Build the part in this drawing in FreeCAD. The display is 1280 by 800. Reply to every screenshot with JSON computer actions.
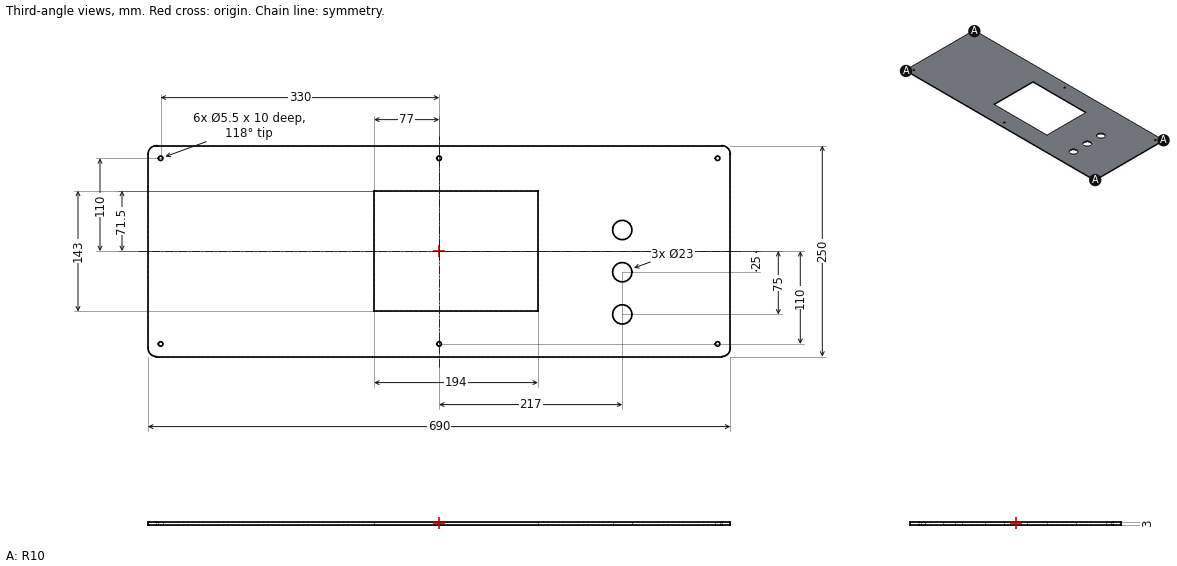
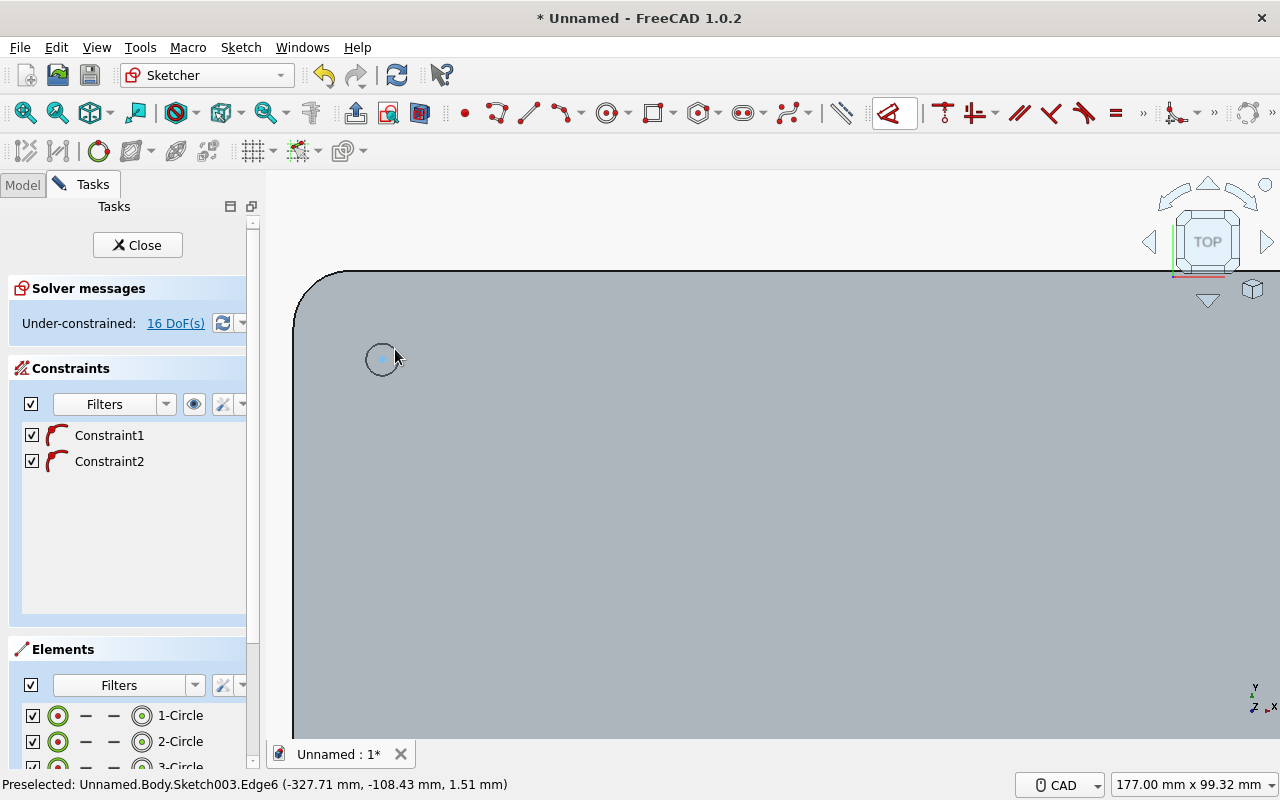
{"action": "left_click", "coordinate": [394, 348]}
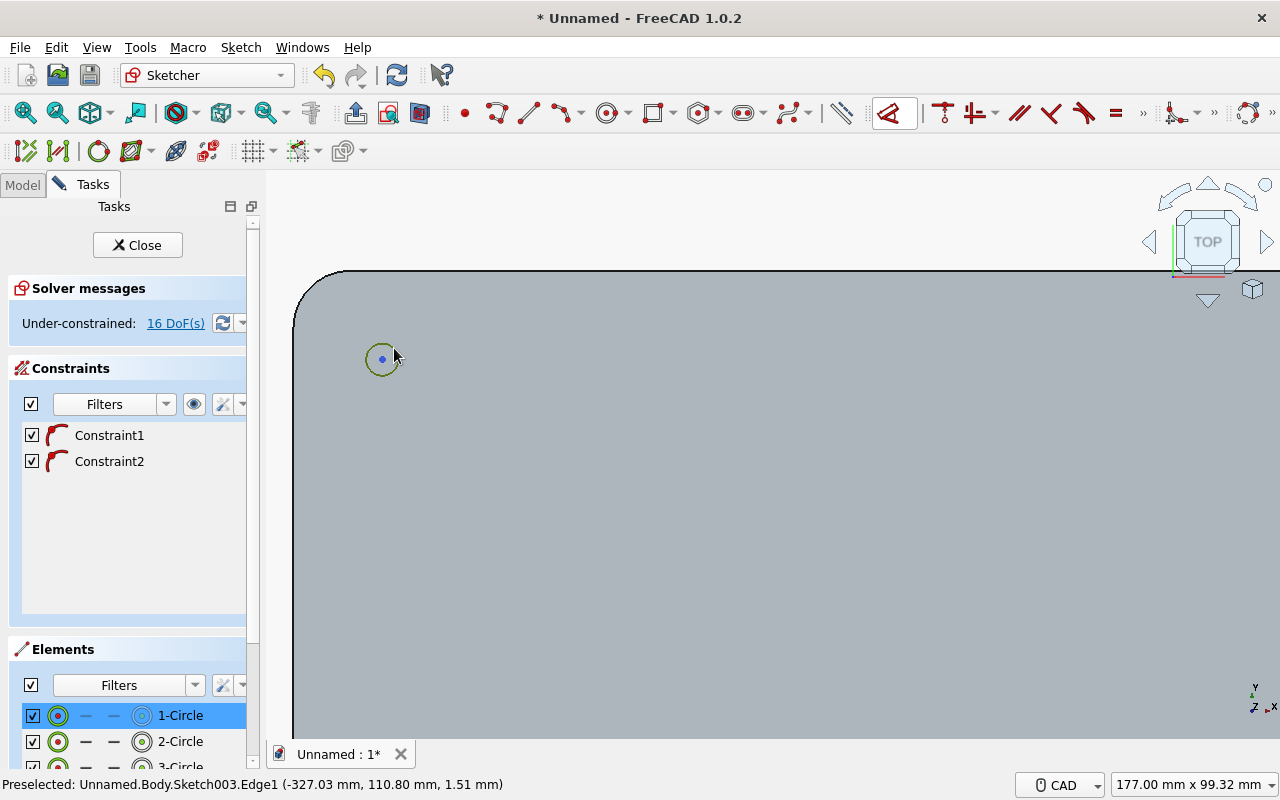
{"action": "scroll", "coordinate": [395, 349], "scroll_direction": "down", "scroll_amount": 9}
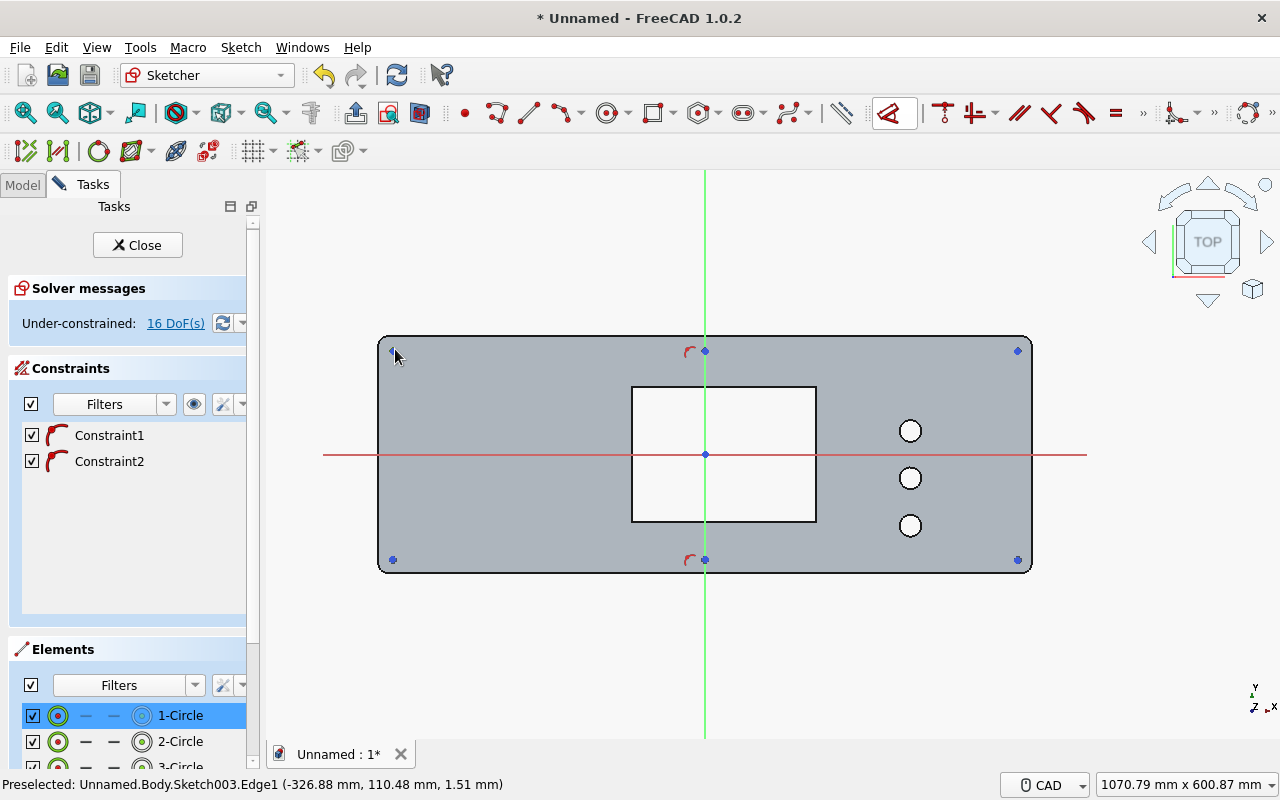
{"action": "scroll", "coordinate": [707, 349], "scroll_direction": "up", "scroll_amount": 10}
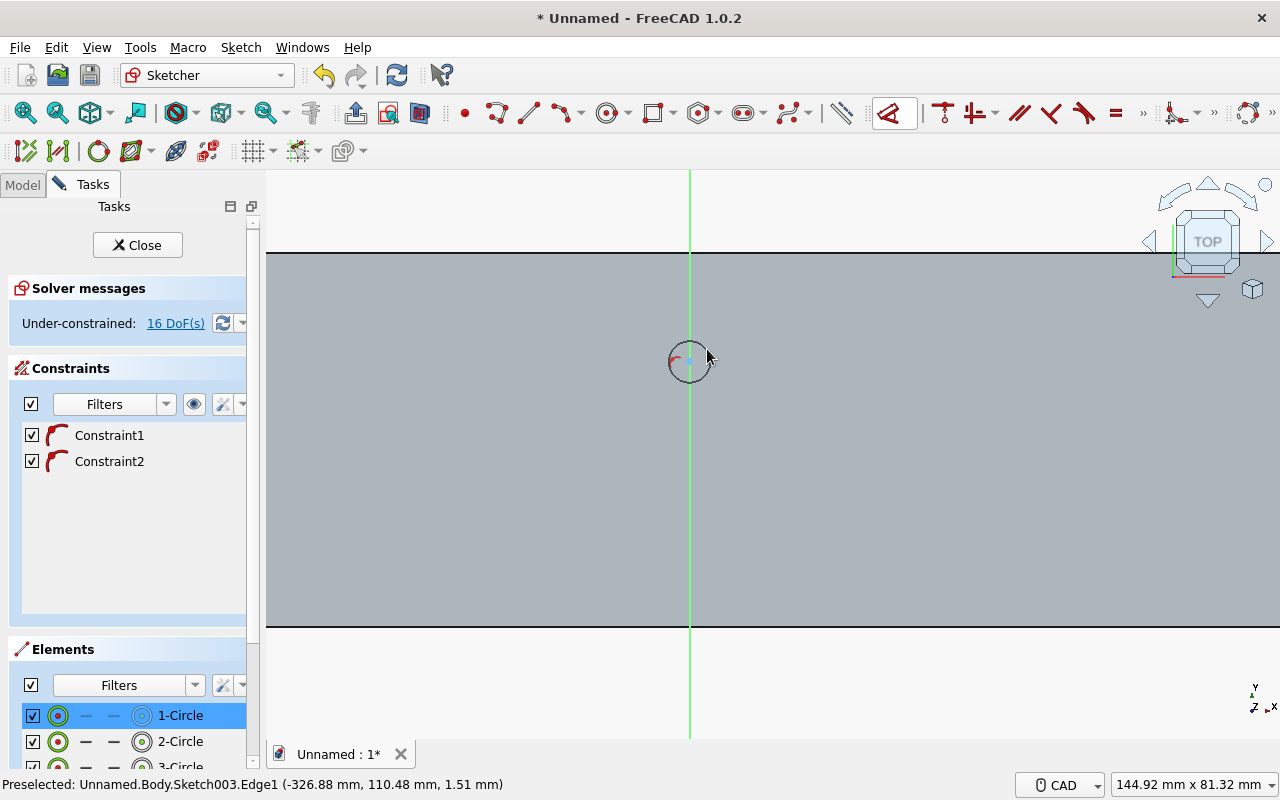
{"action": "left_click", "coordinate": [704, 347]}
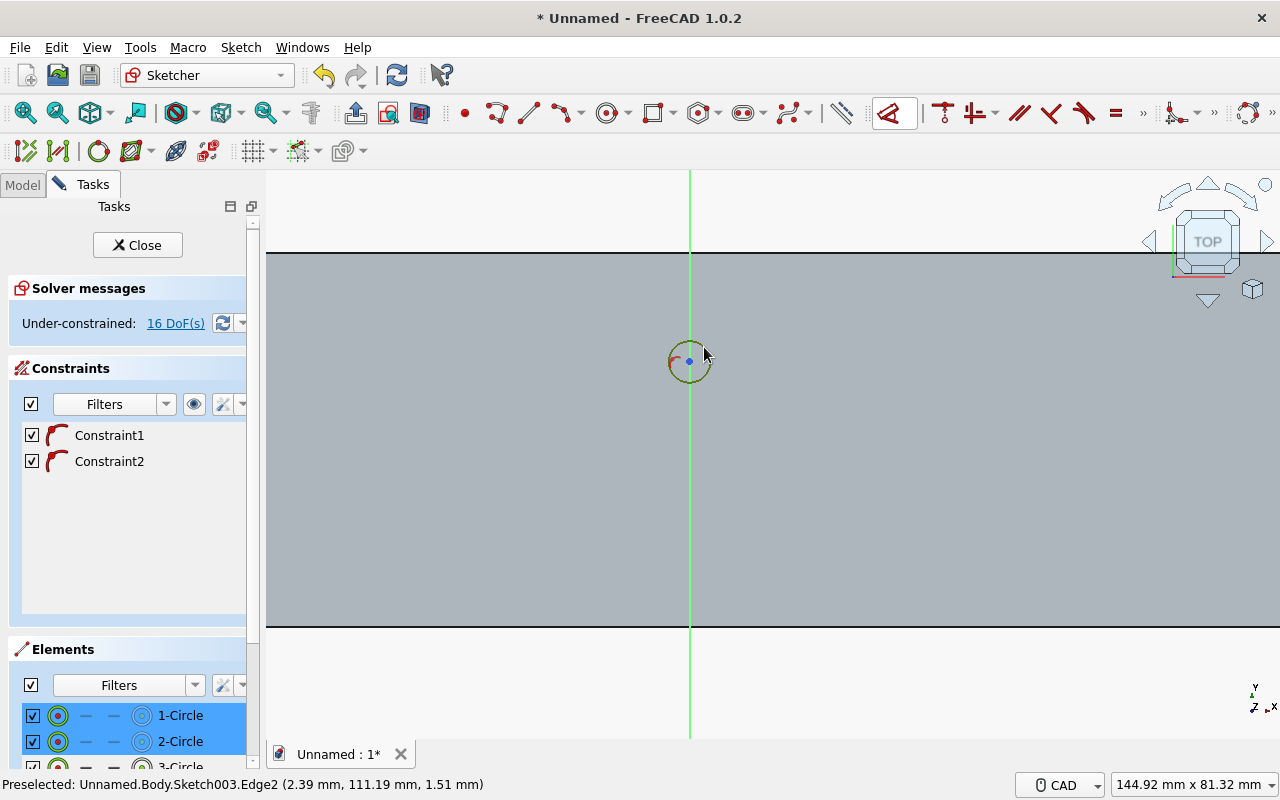
{"action": "scroll", "coordinate": [707, 349], "scroll_direction": "down", "scroll_amount": 10}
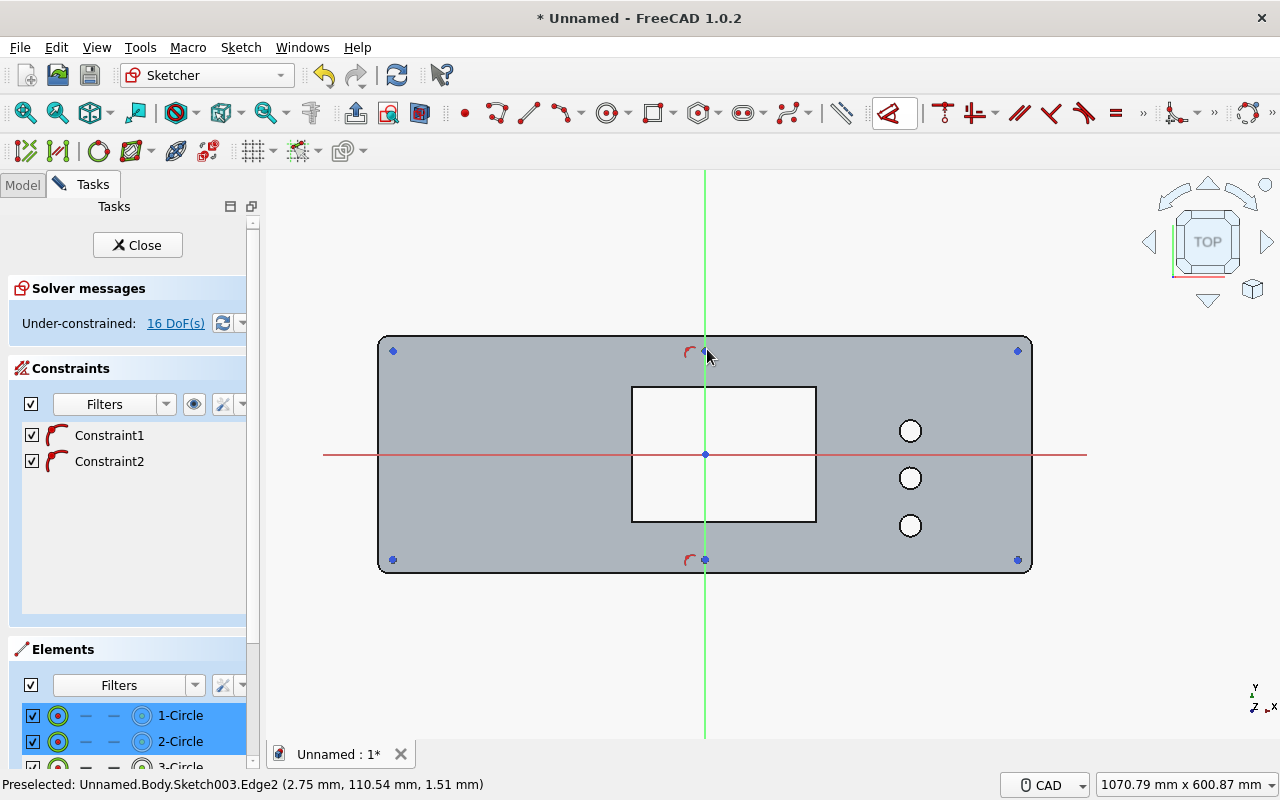
{"action": "scroll", "coordinate": [1020, 349], "scroll_direction": "up", "scroll_amount": 9}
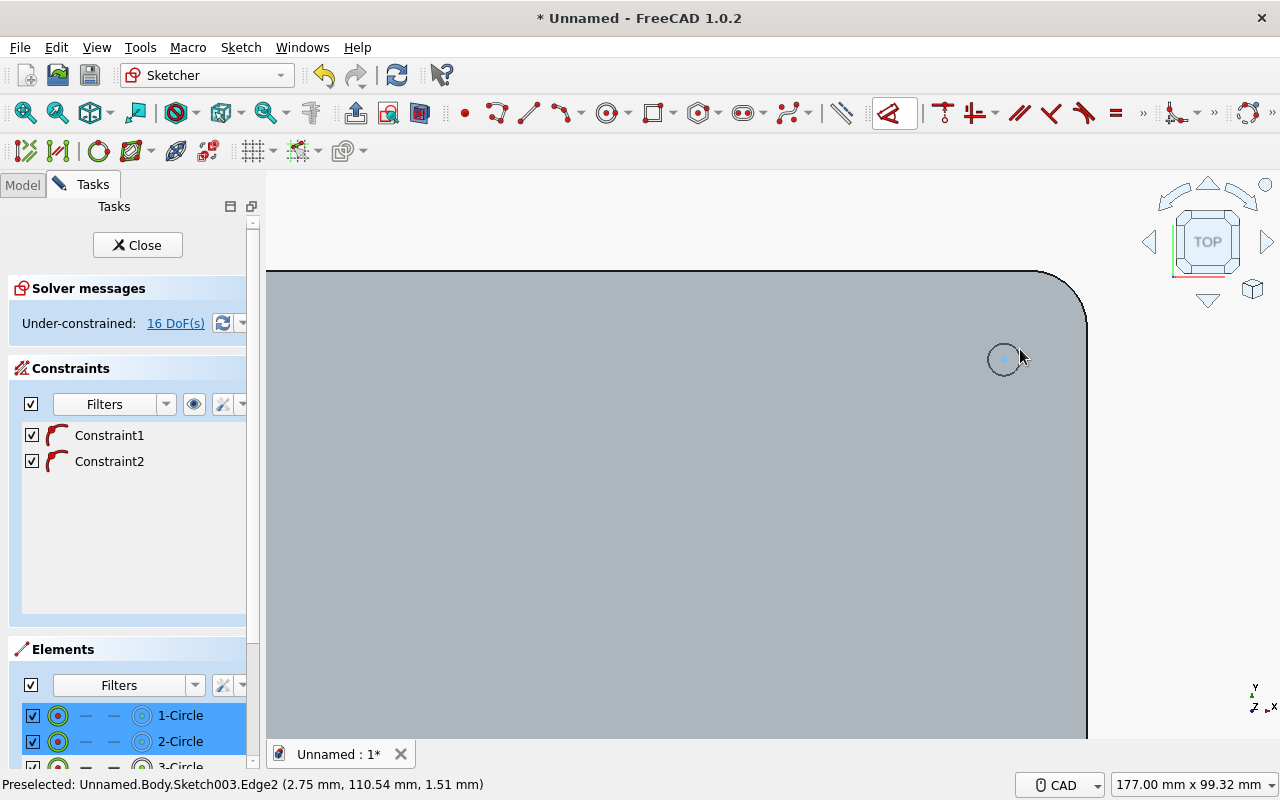
{"action": "left_click", "coordinate": [1015, 348]}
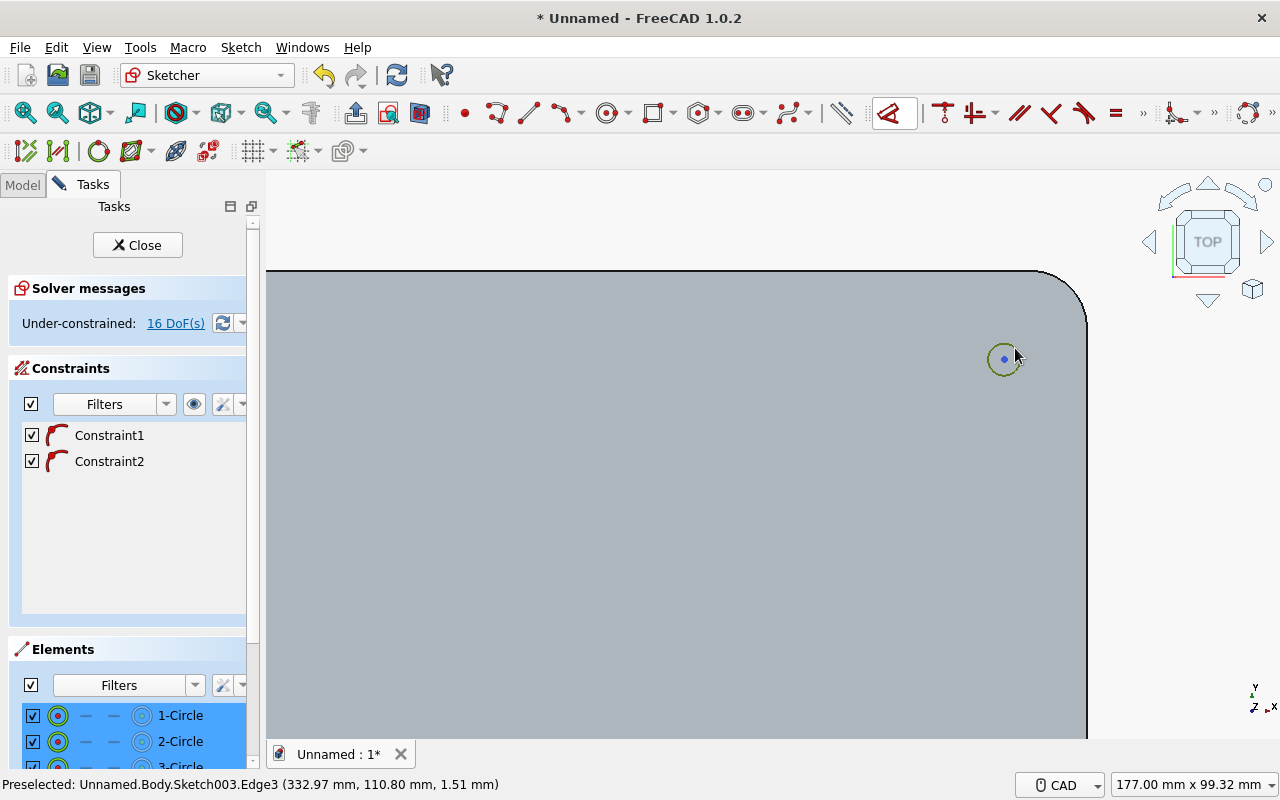
{"action": "scroll", "coordinate": [1020, 349], "scroll_direction": "down", "scroll_amount": 9}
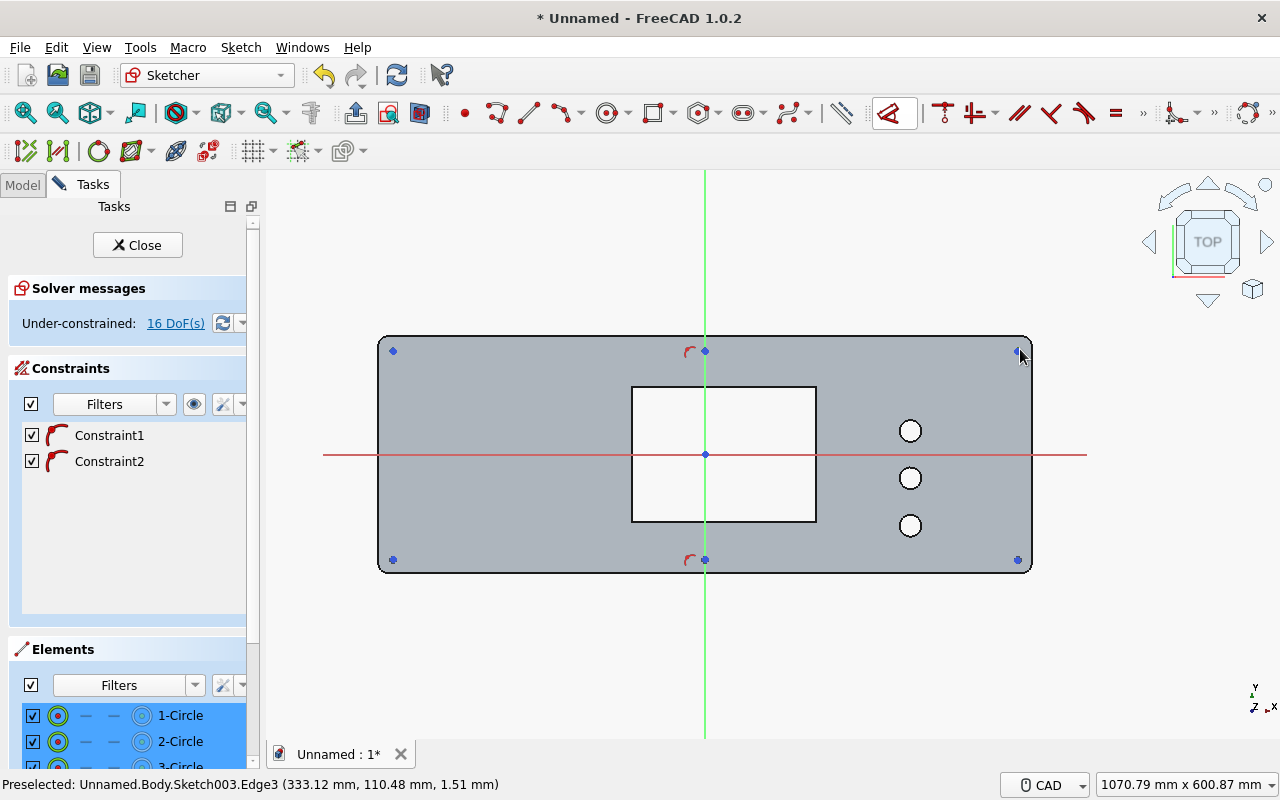
{"action": "scroll", "coordinate": [1020, 558], "scroll_direction": "up", "scroll_amount": 8}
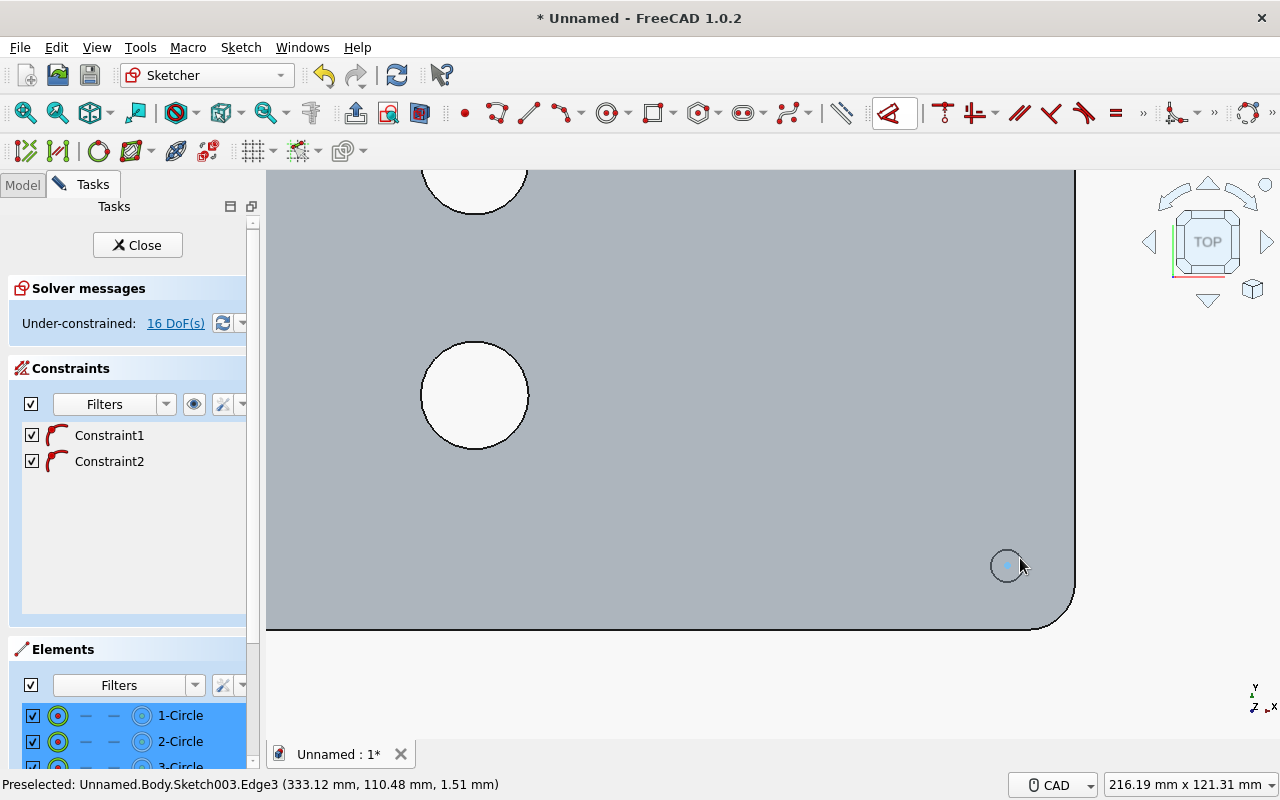
{"action": "left_click", "coordinate": [1019, 554]}